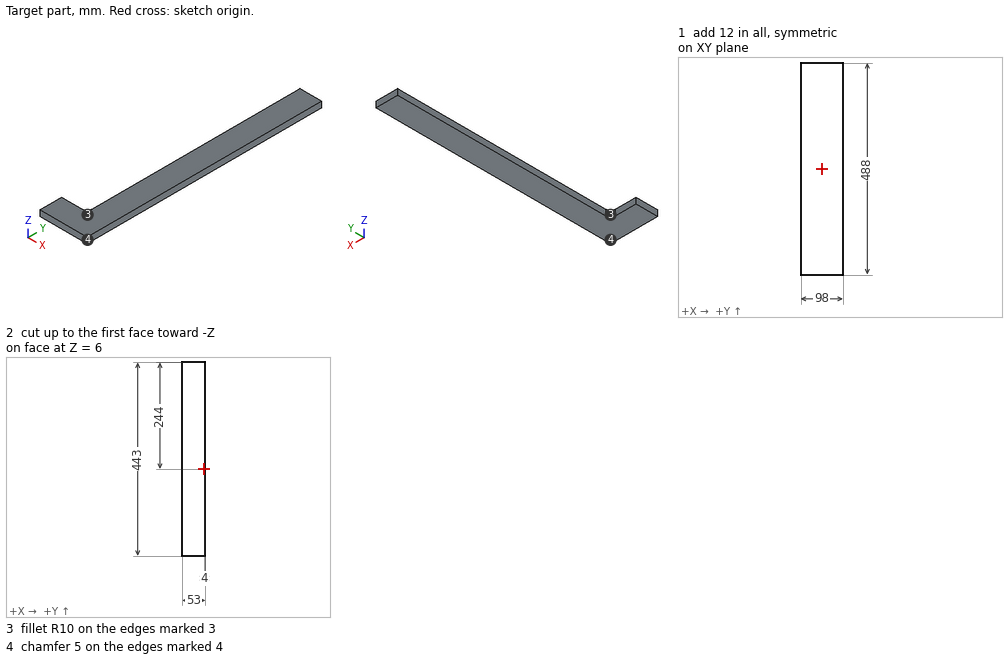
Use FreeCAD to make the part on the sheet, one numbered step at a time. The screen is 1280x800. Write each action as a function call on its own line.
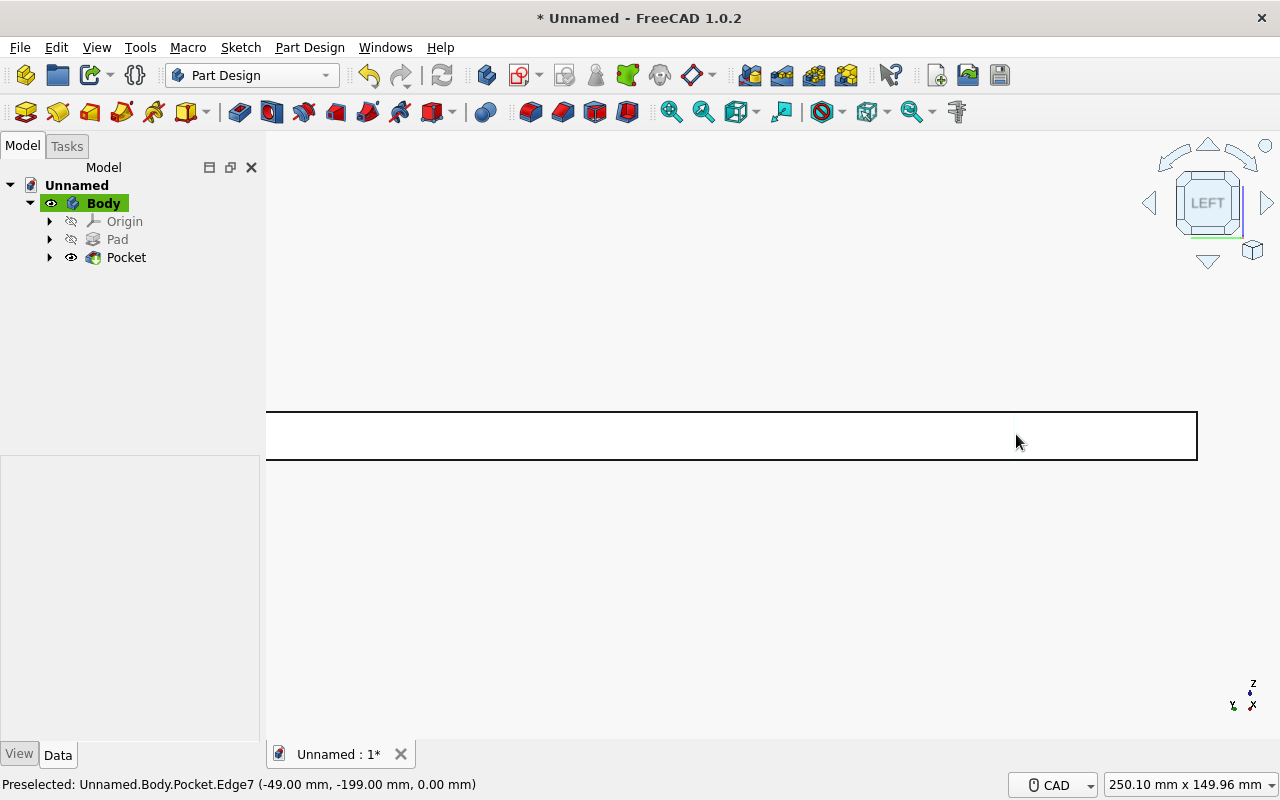
click(672, 112)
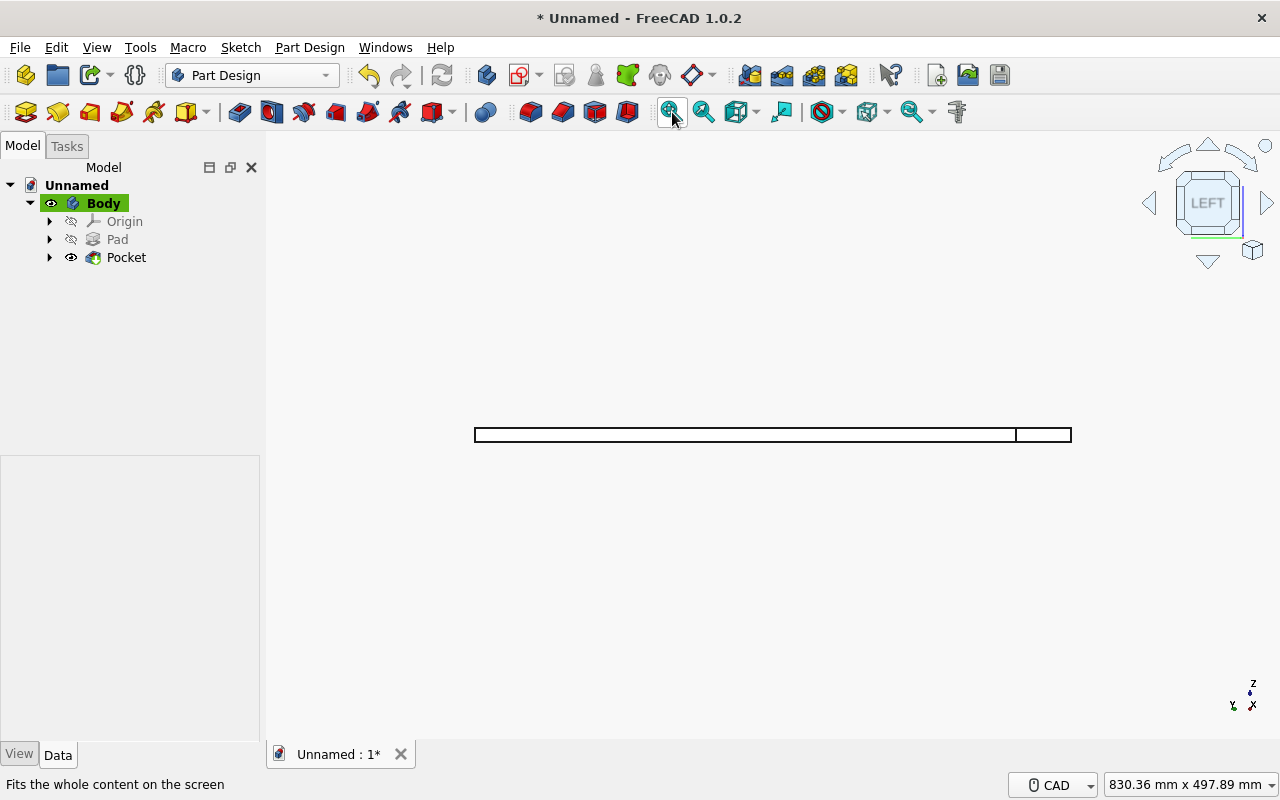
key(v)
key(3)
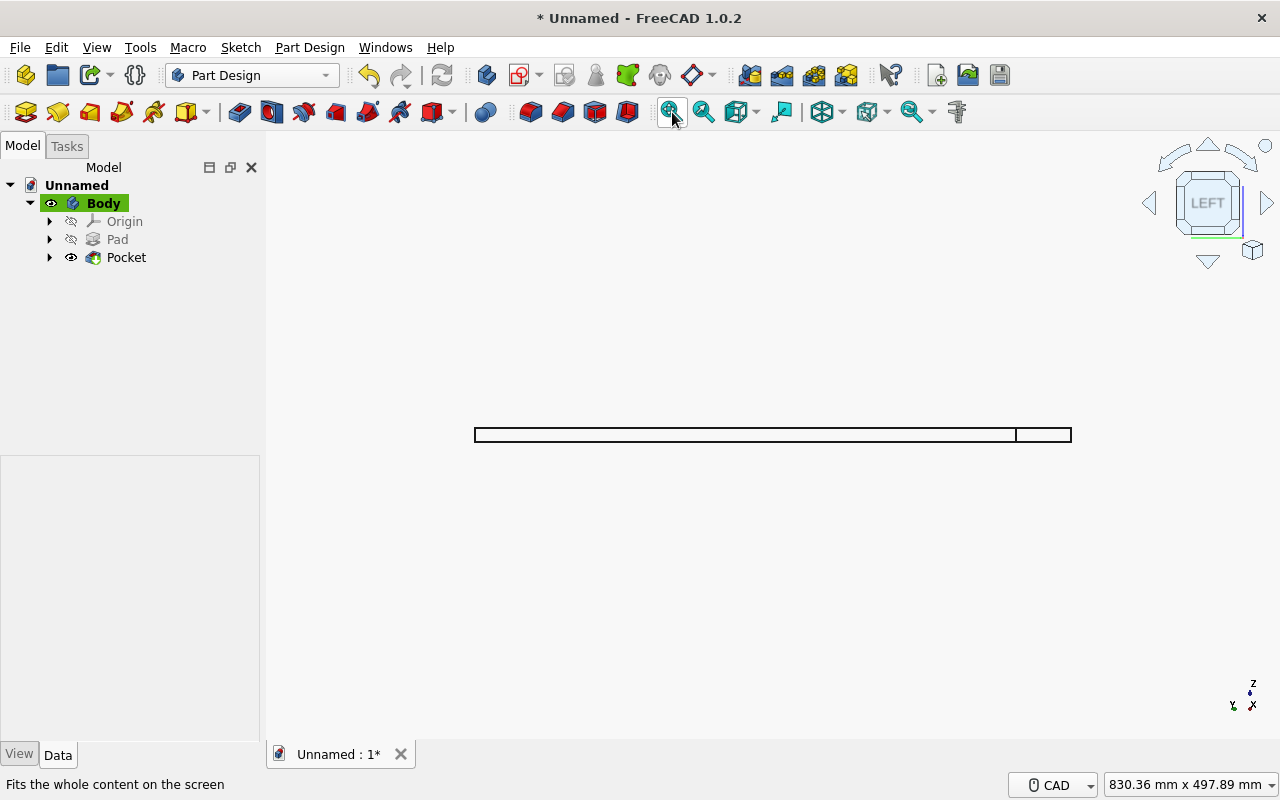
key(0)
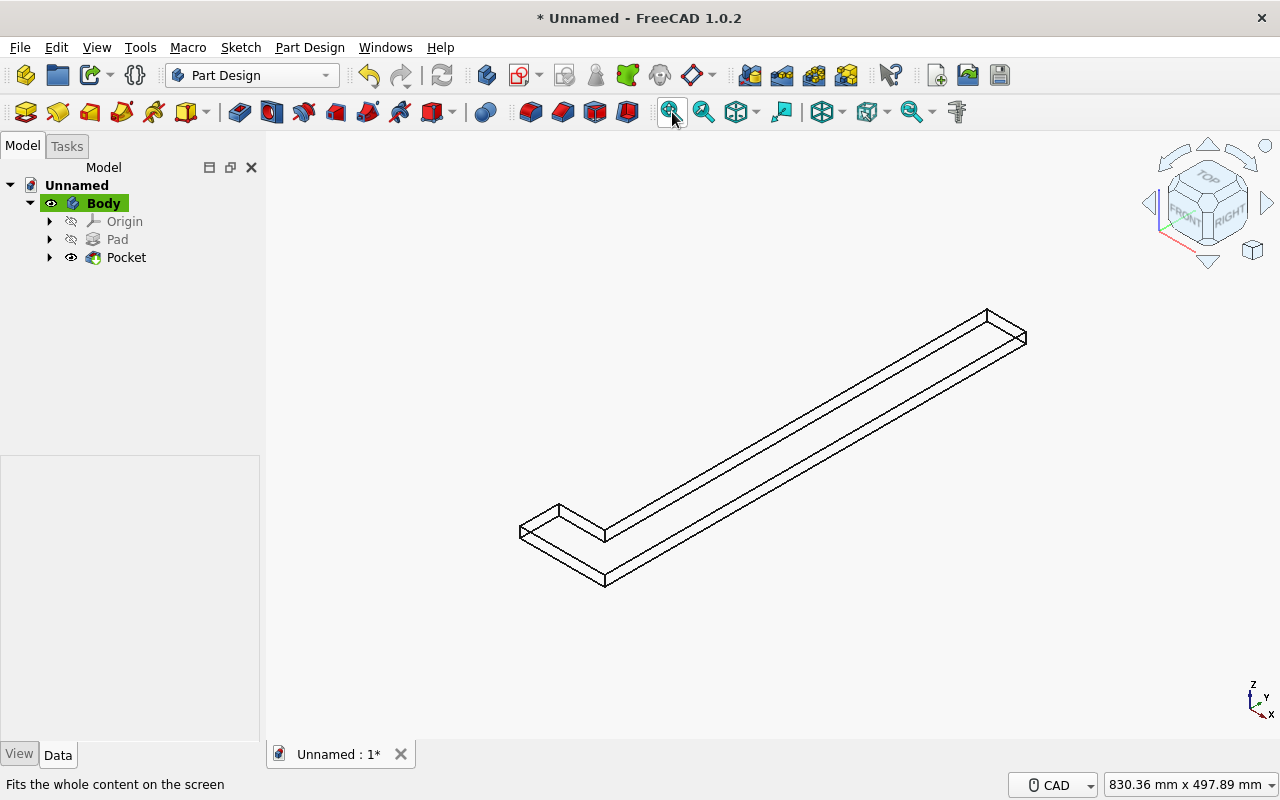
click(605, 536)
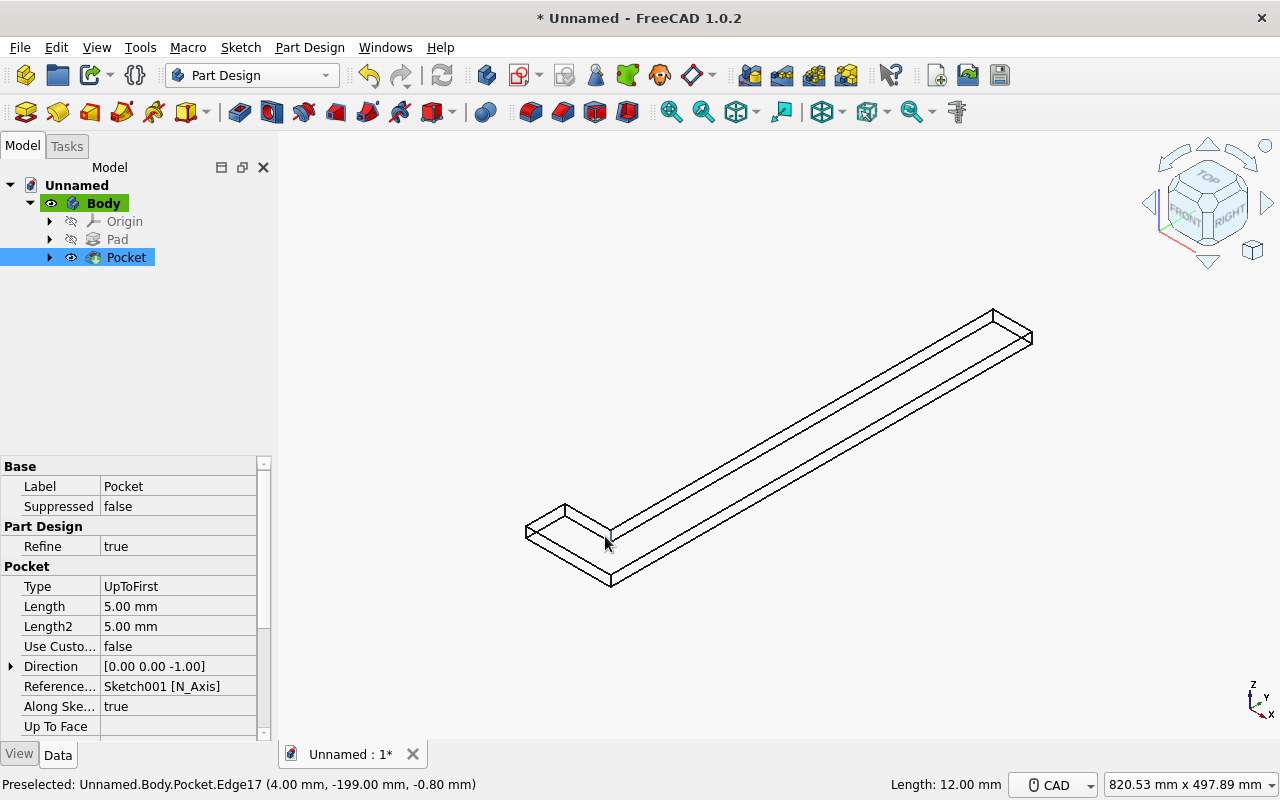
key(v)
key(1)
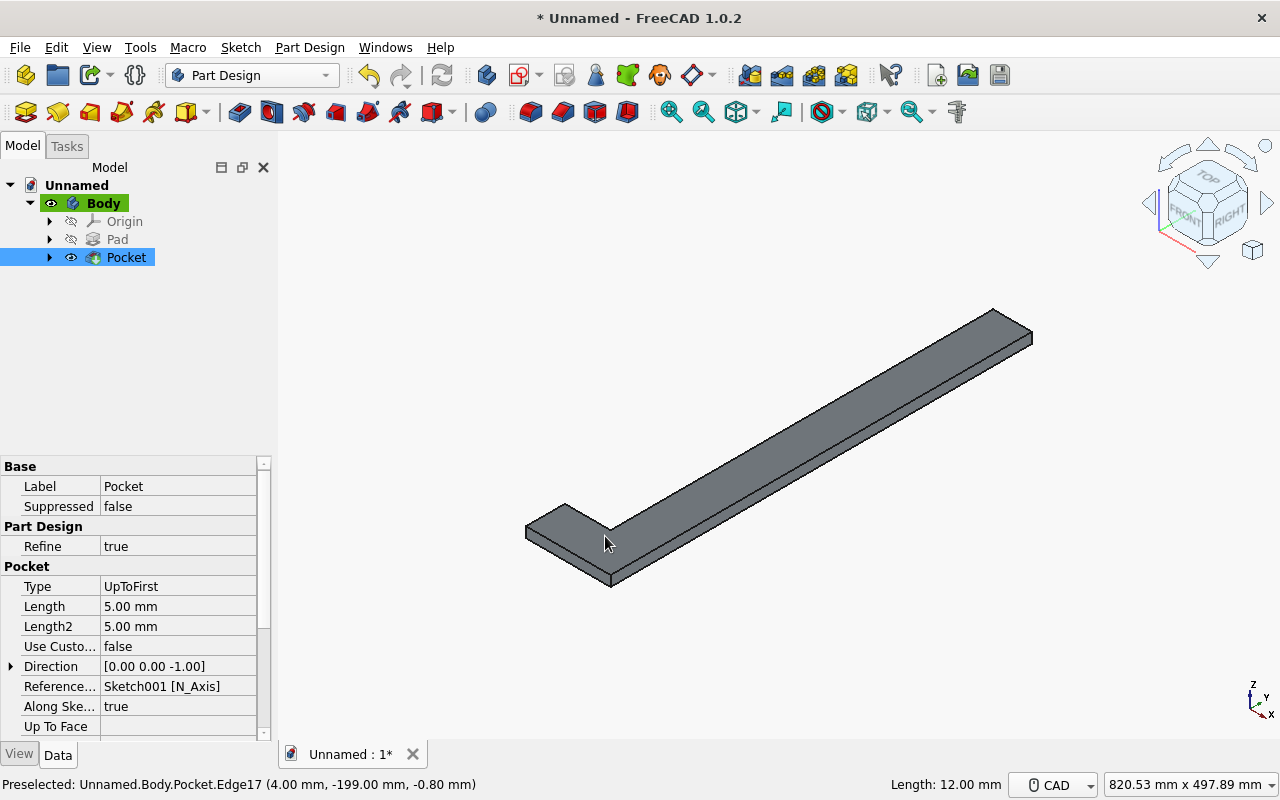
click(532, 112)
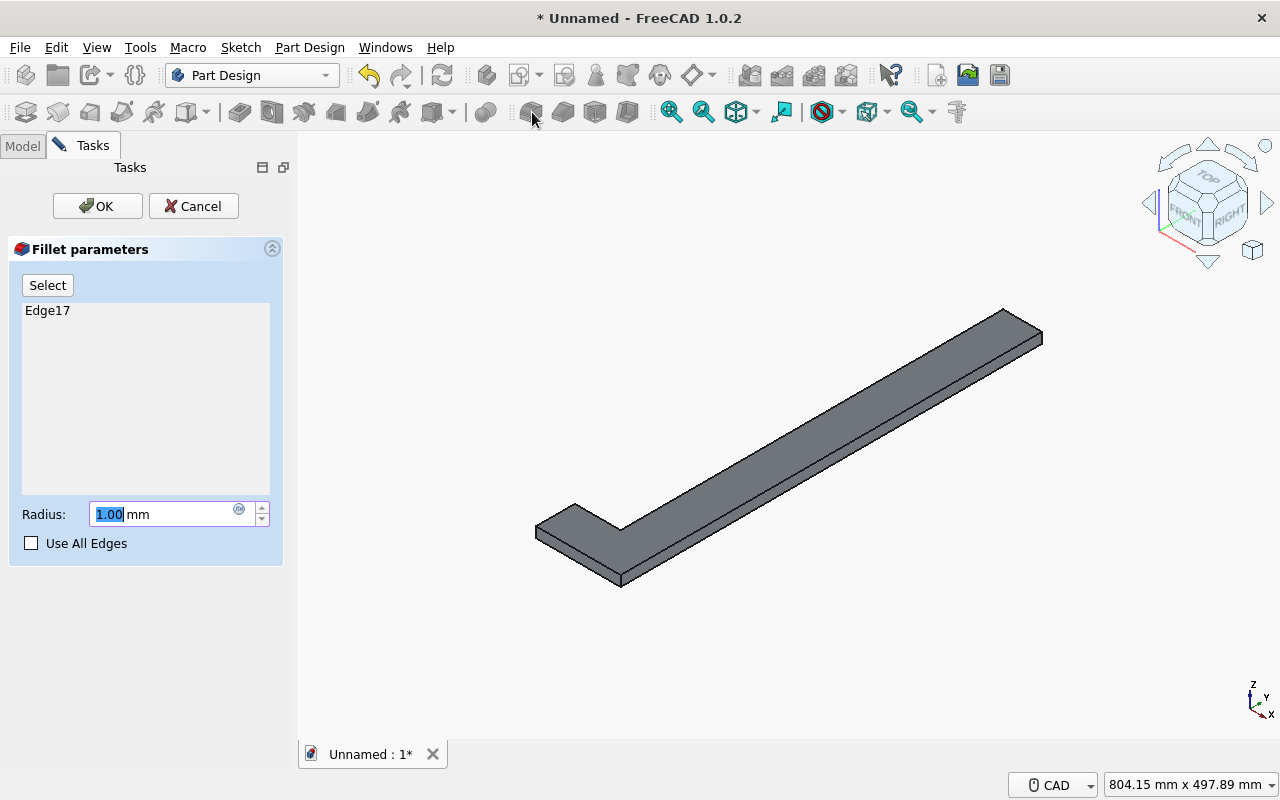
text(10)
key(Tab)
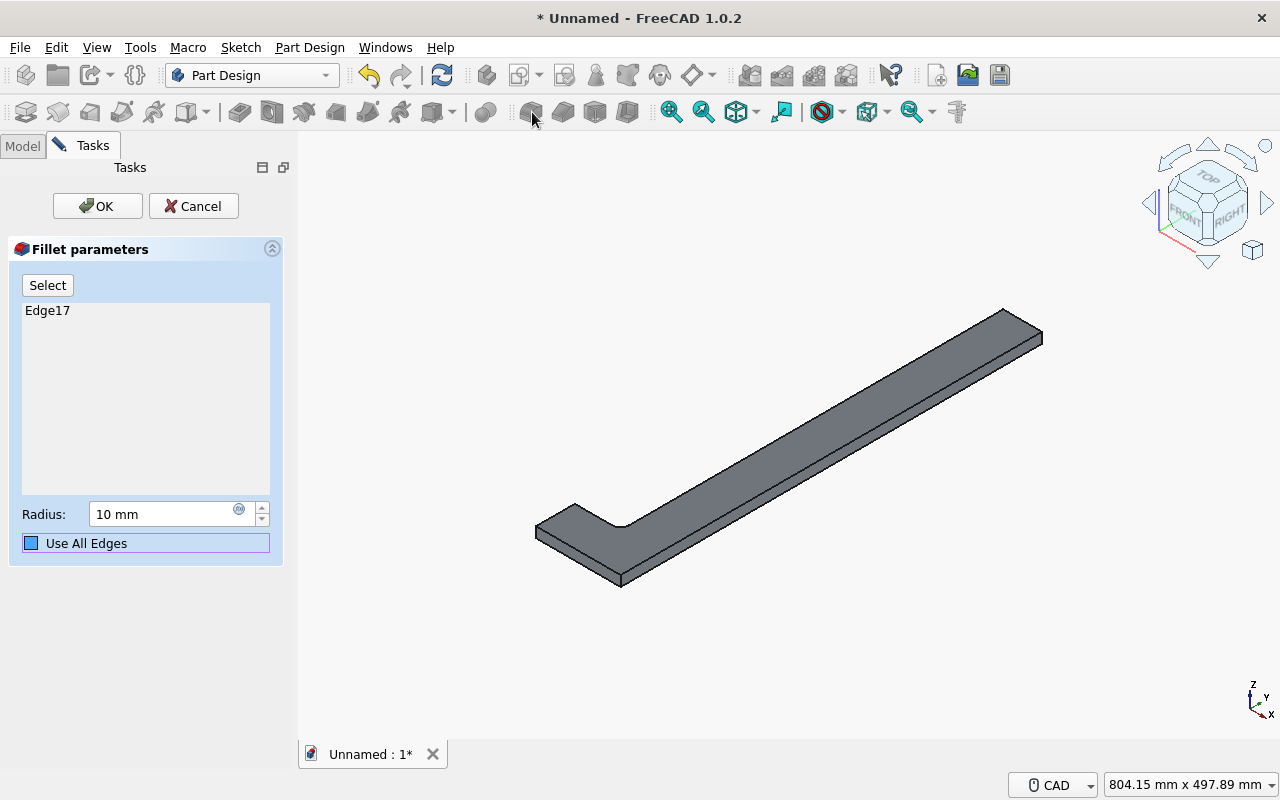
click(98, 206)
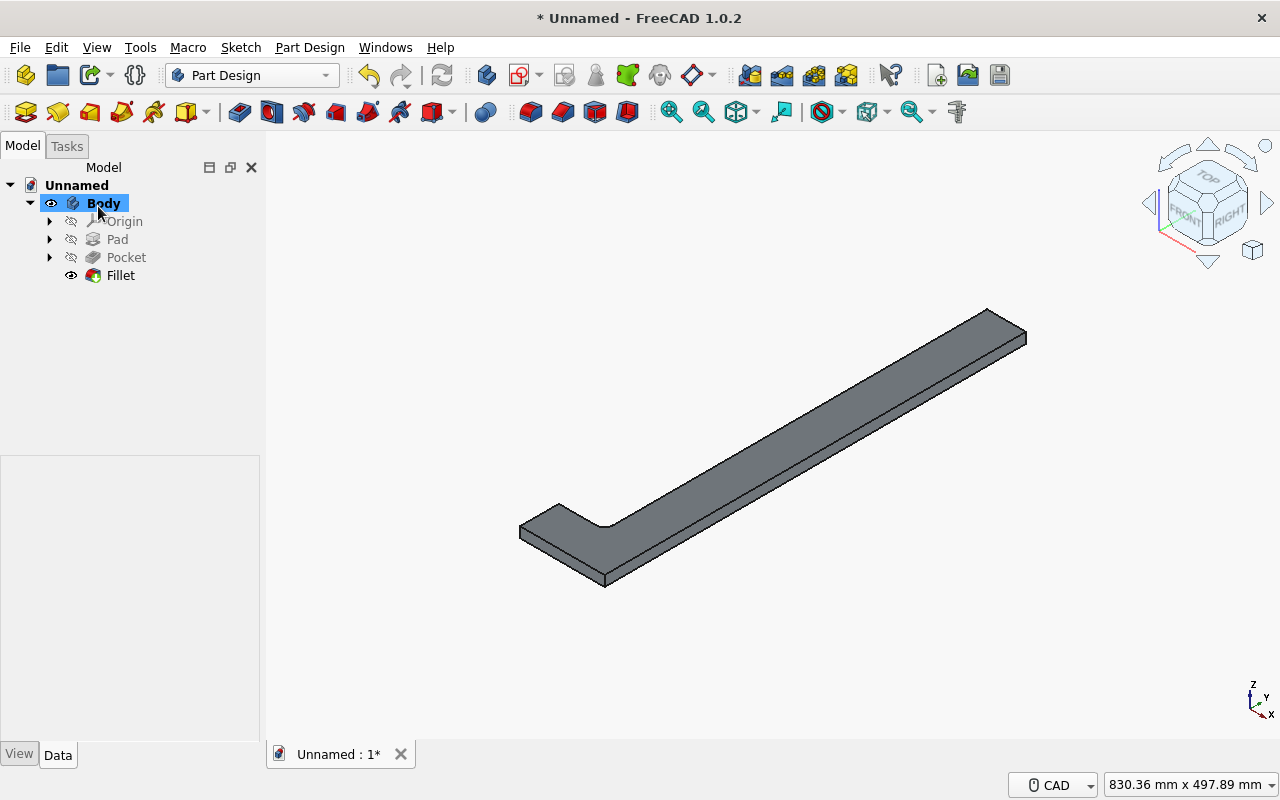
click(605, 581)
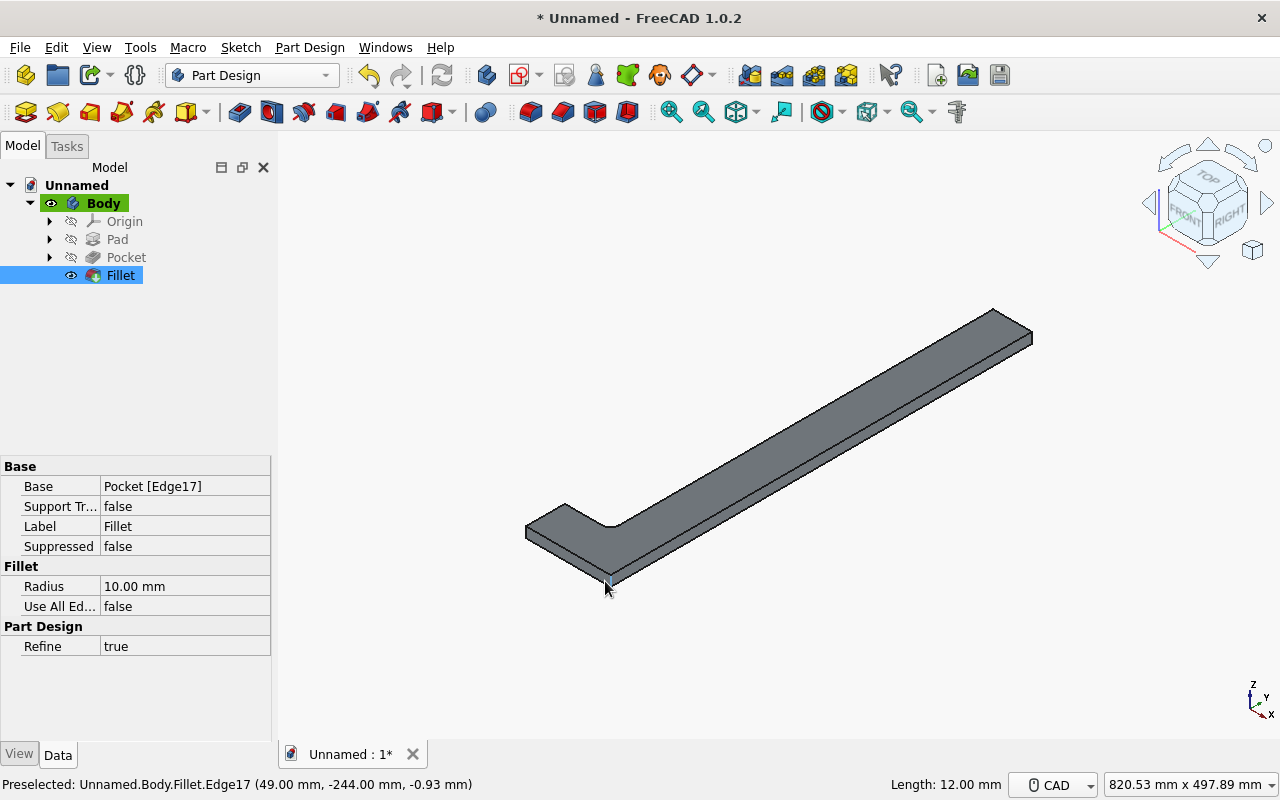
click(564, 112)